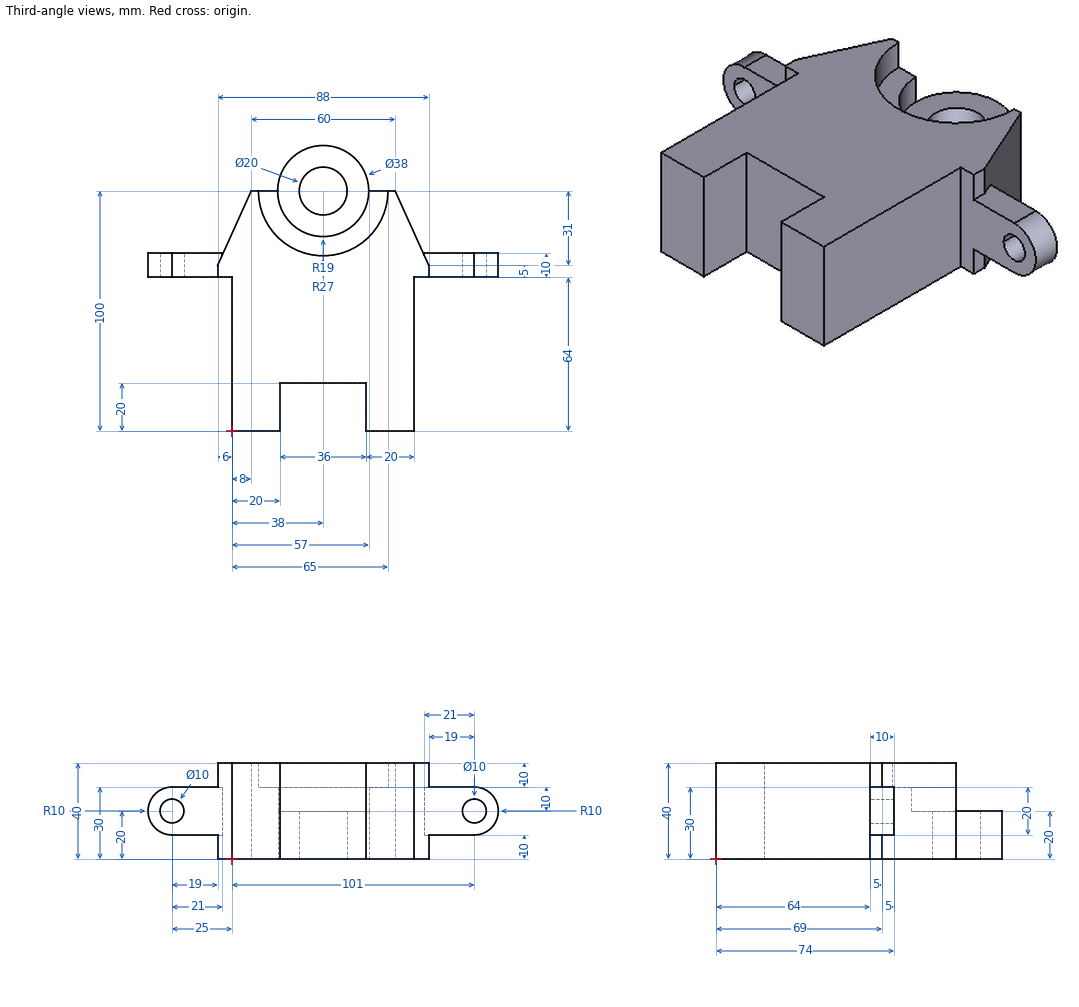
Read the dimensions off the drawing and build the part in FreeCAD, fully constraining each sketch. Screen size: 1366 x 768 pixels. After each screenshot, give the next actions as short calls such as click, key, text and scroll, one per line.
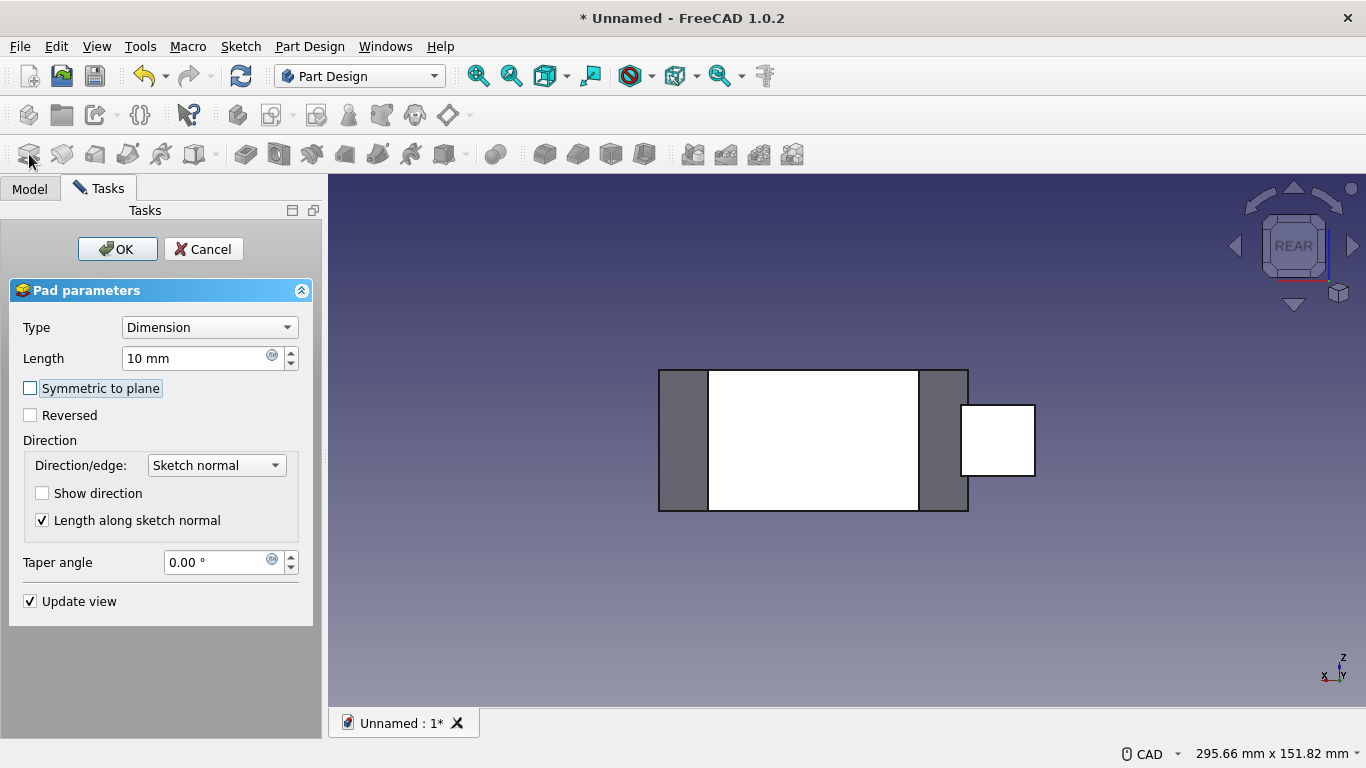
click(31, 415)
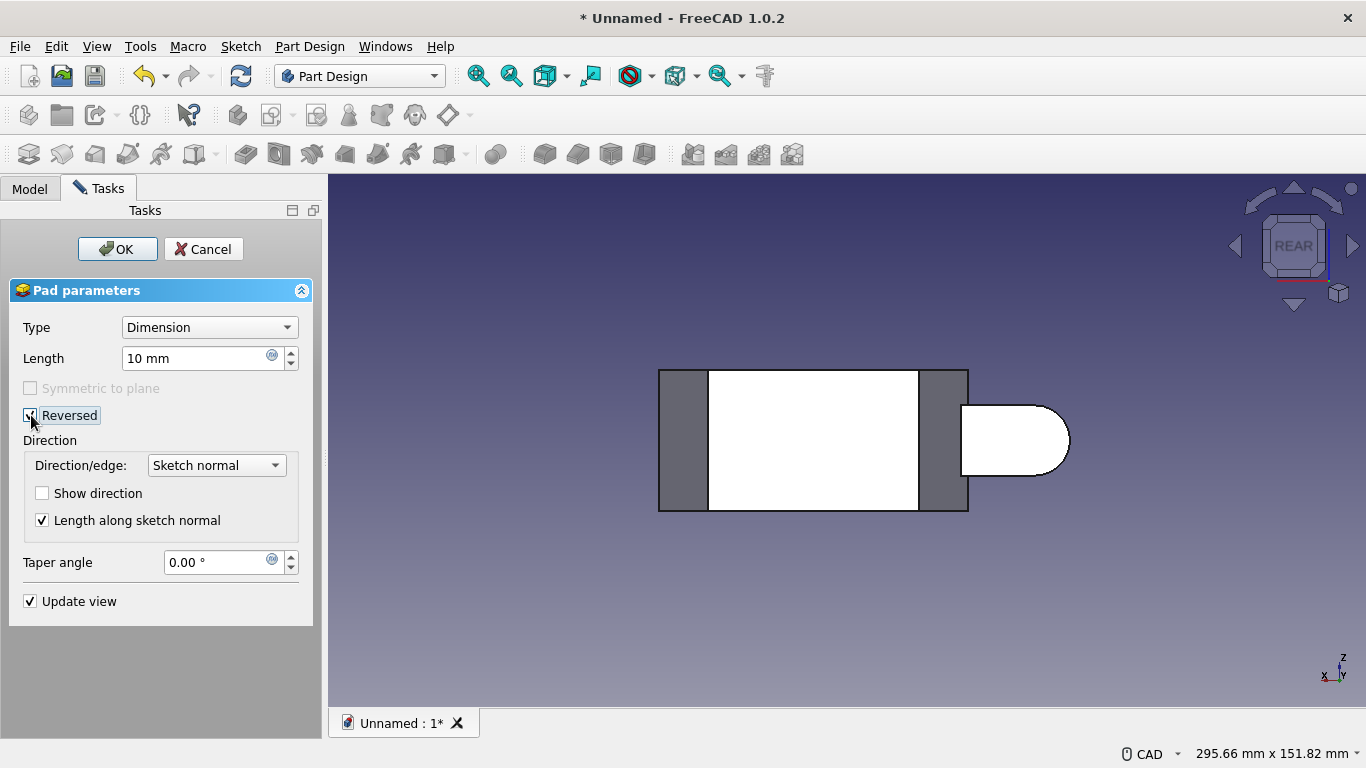
click(118, 249)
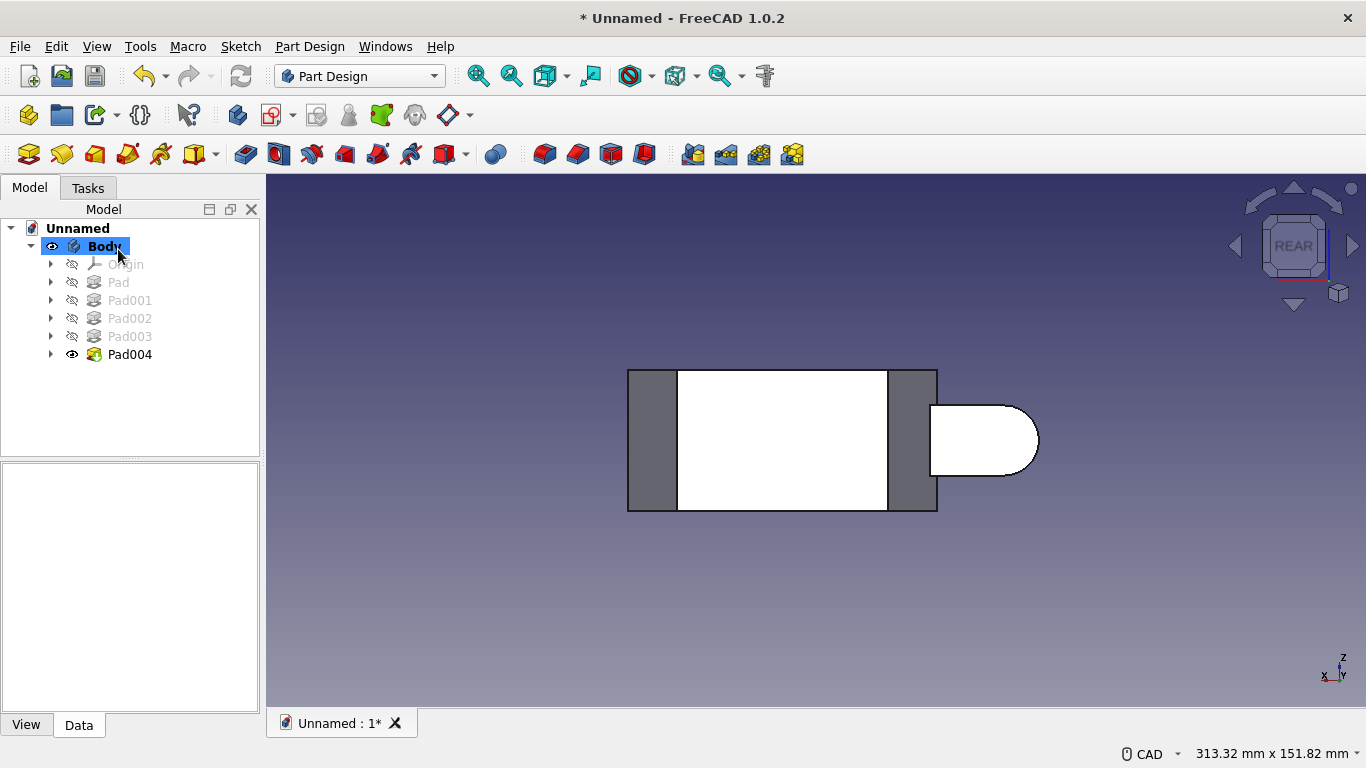
click(479, 76)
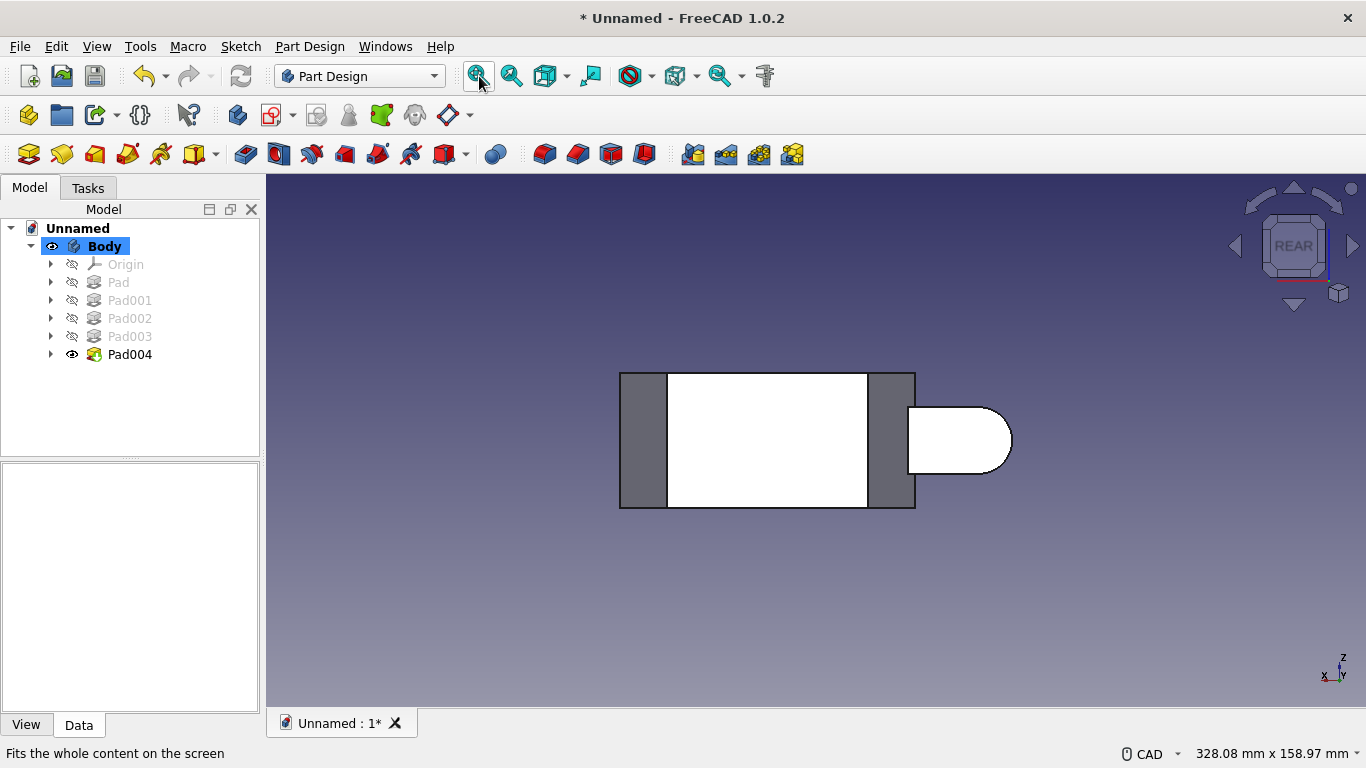
click(945, 439)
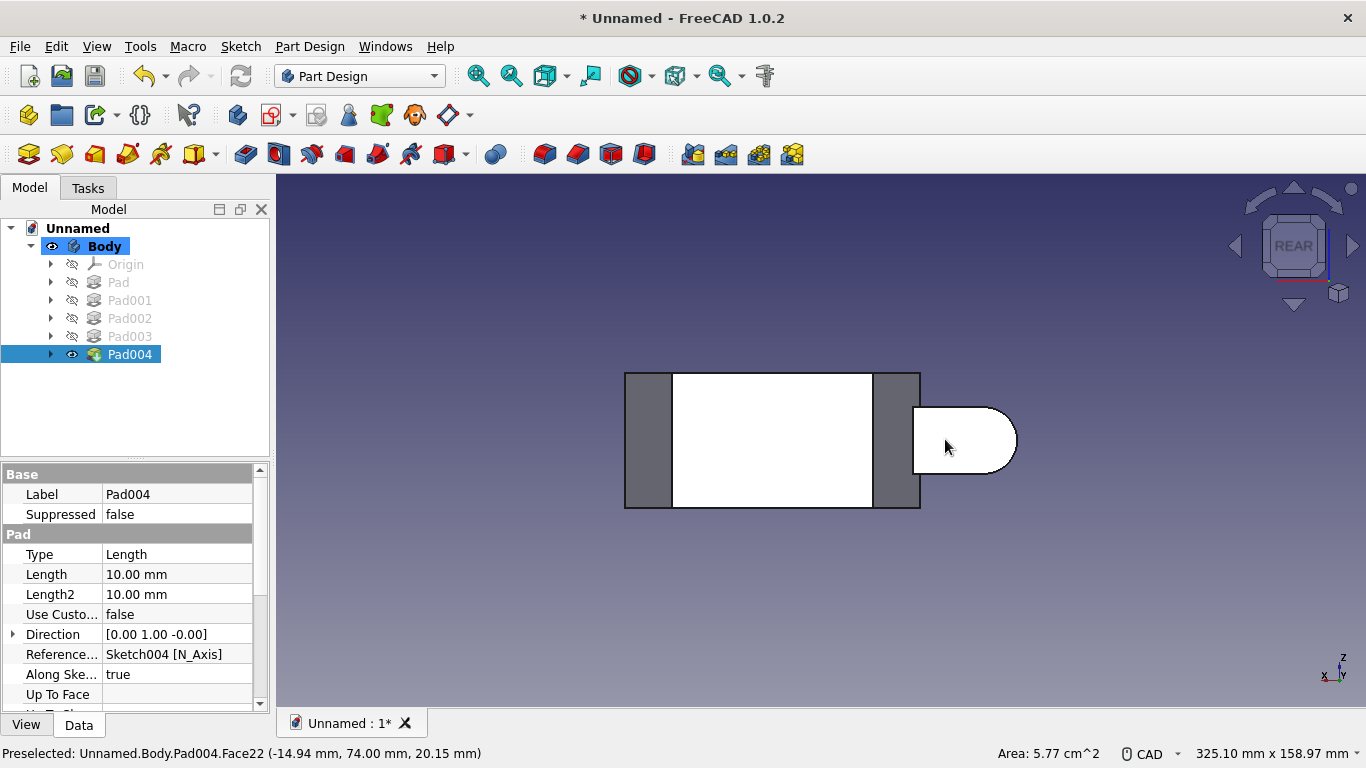
click(270, 116)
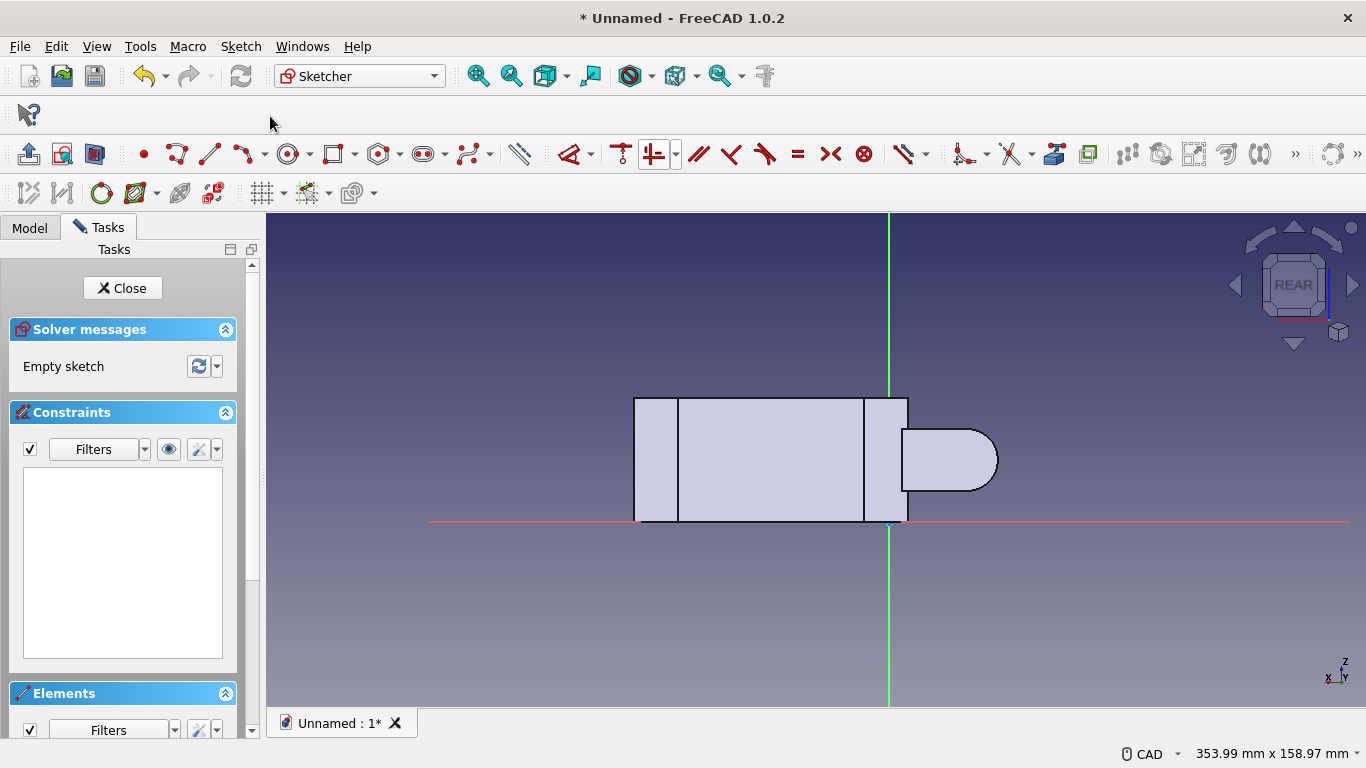
click(95, 154)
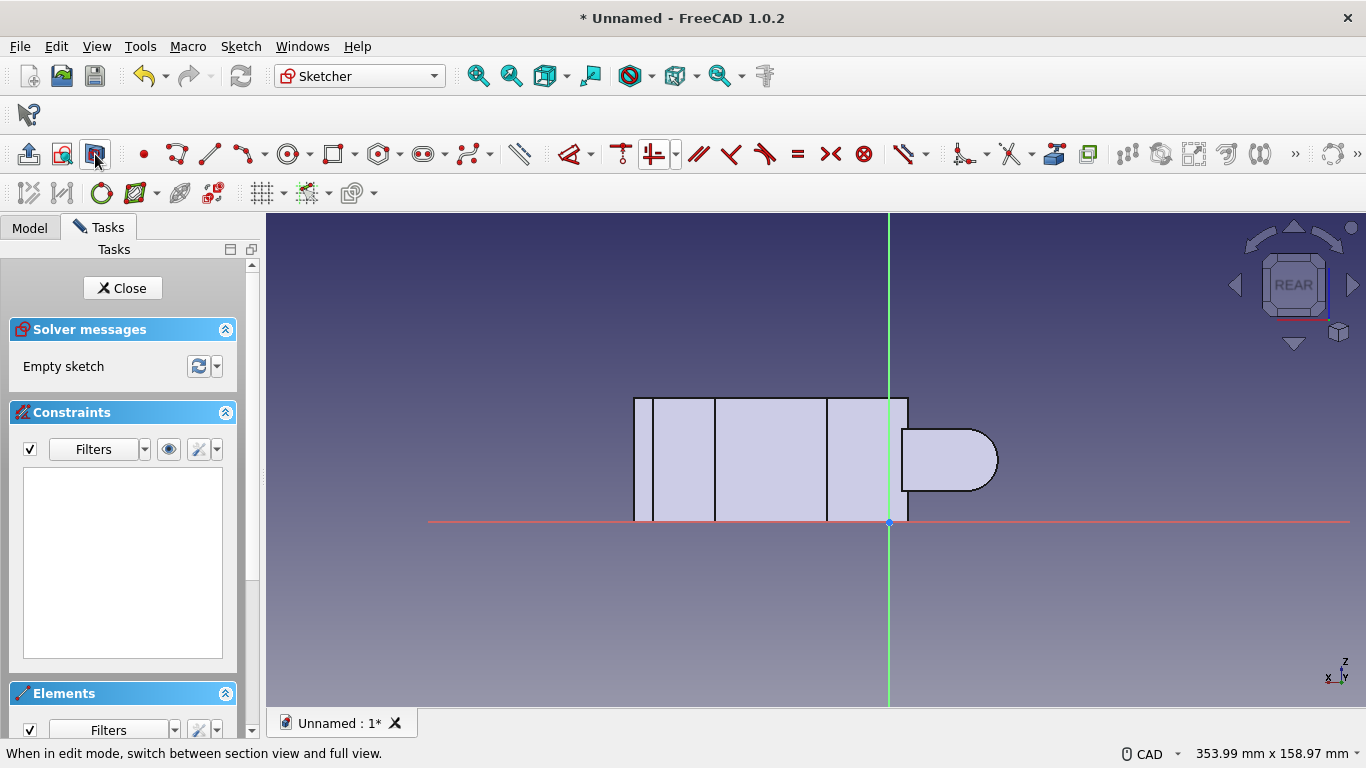
scroll(994, 460, up, 11)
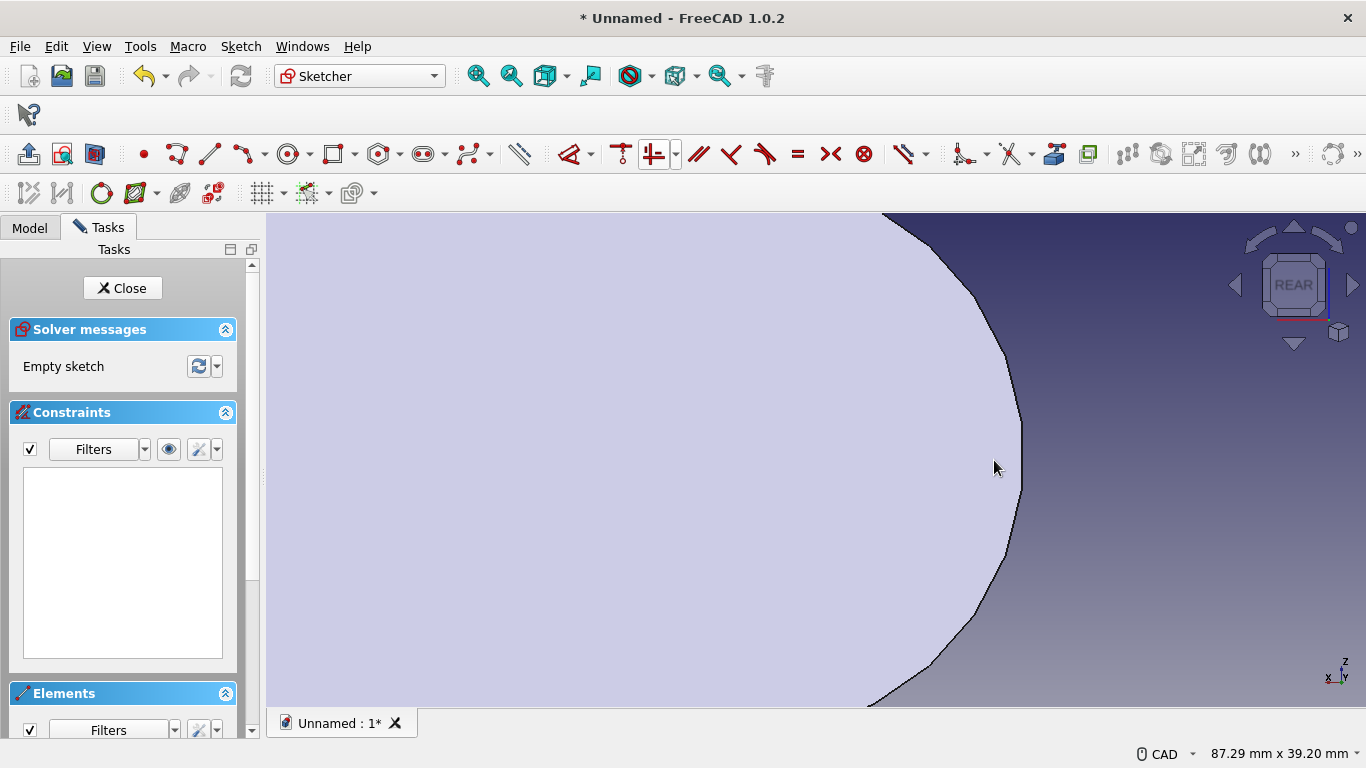
click(288, 154)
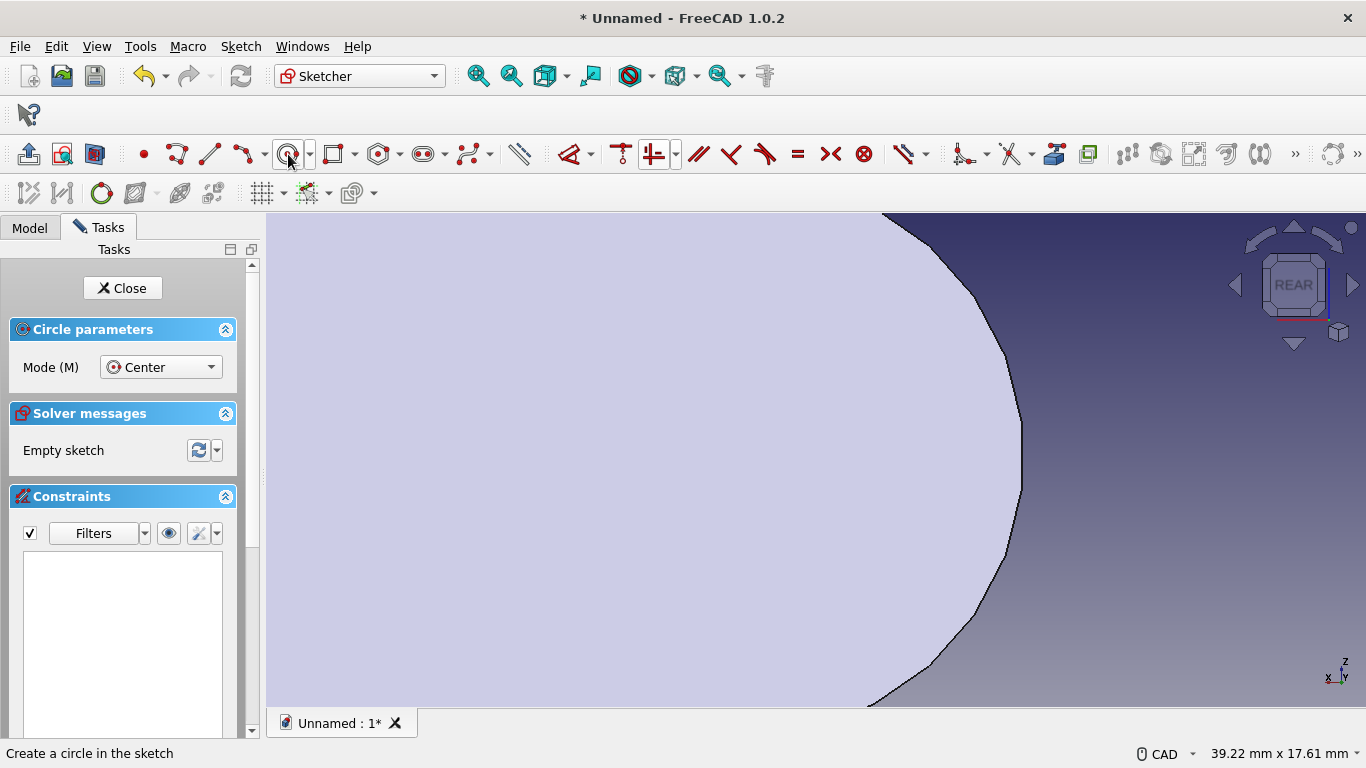
click(743, 456)
click(843, 357)
key(Escape)